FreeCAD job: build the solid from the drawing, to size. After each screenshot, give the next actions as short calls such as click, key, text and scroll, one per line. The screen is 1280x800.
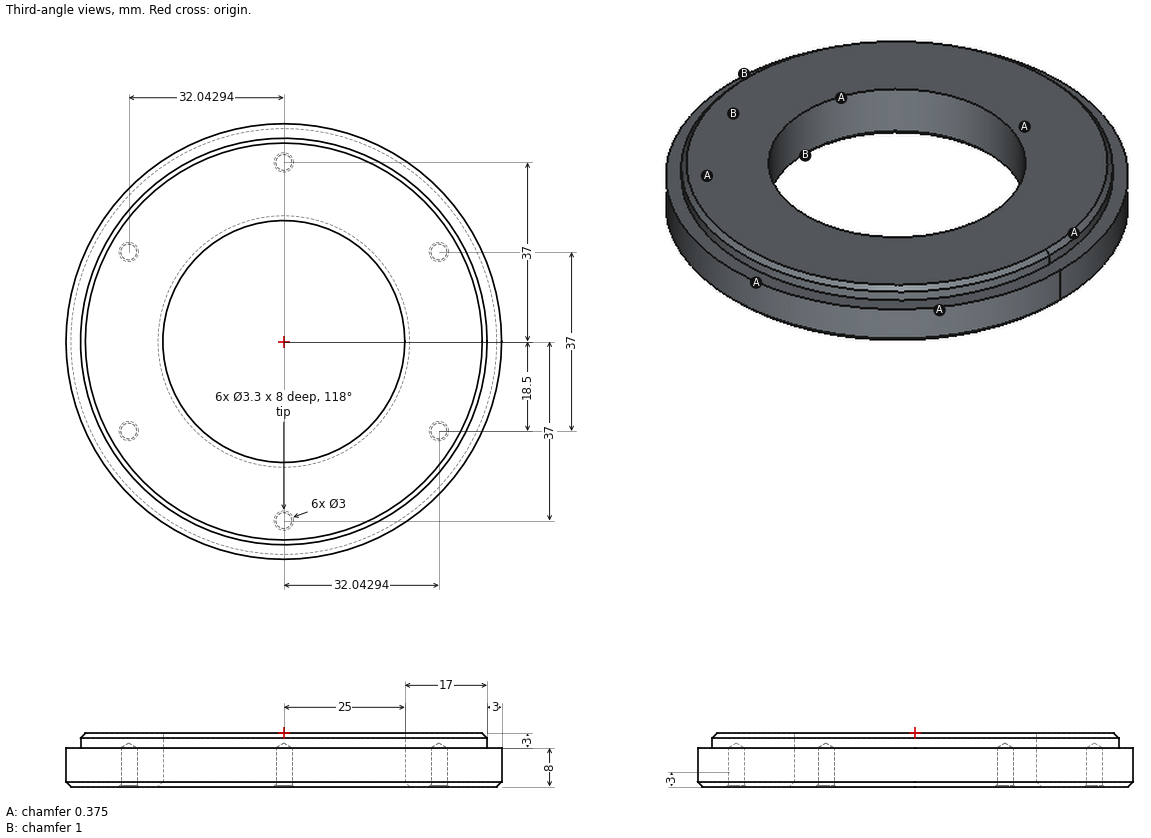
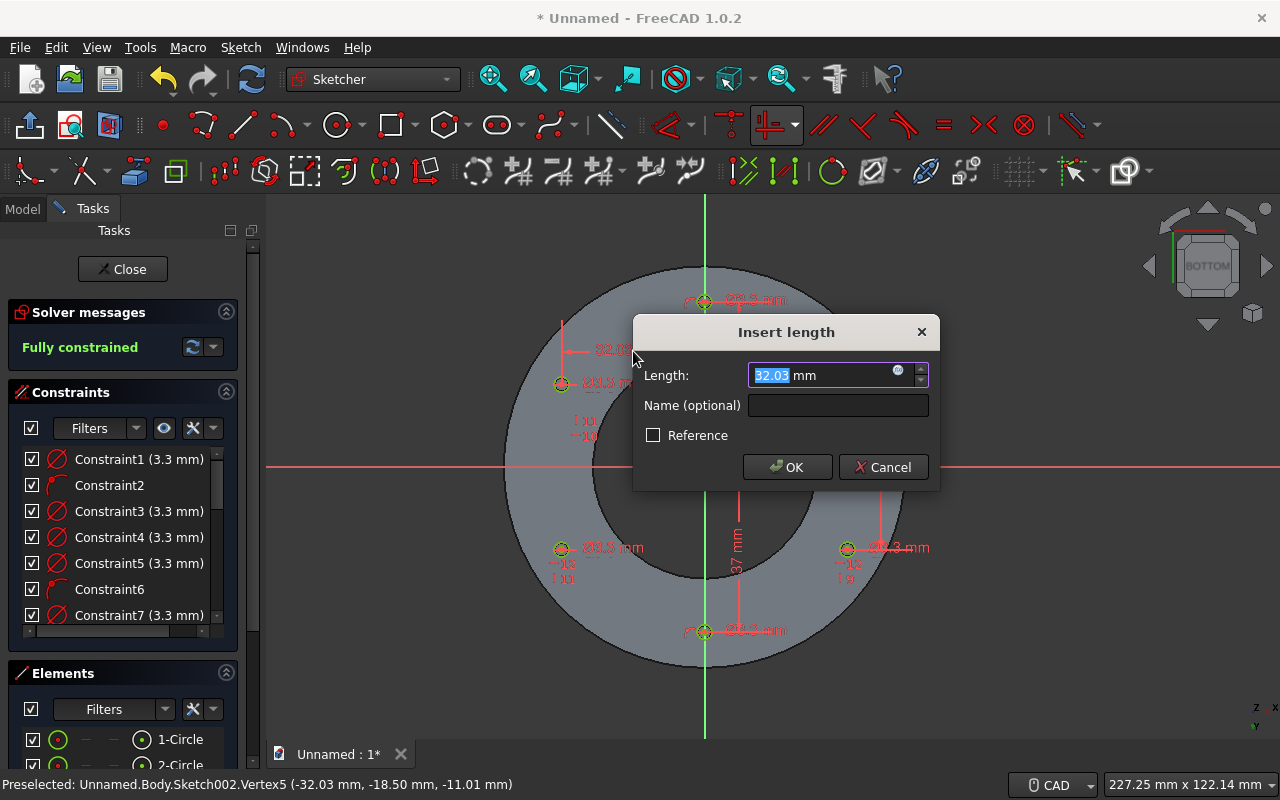
text(32.04294)
key(Return)
key(Escape)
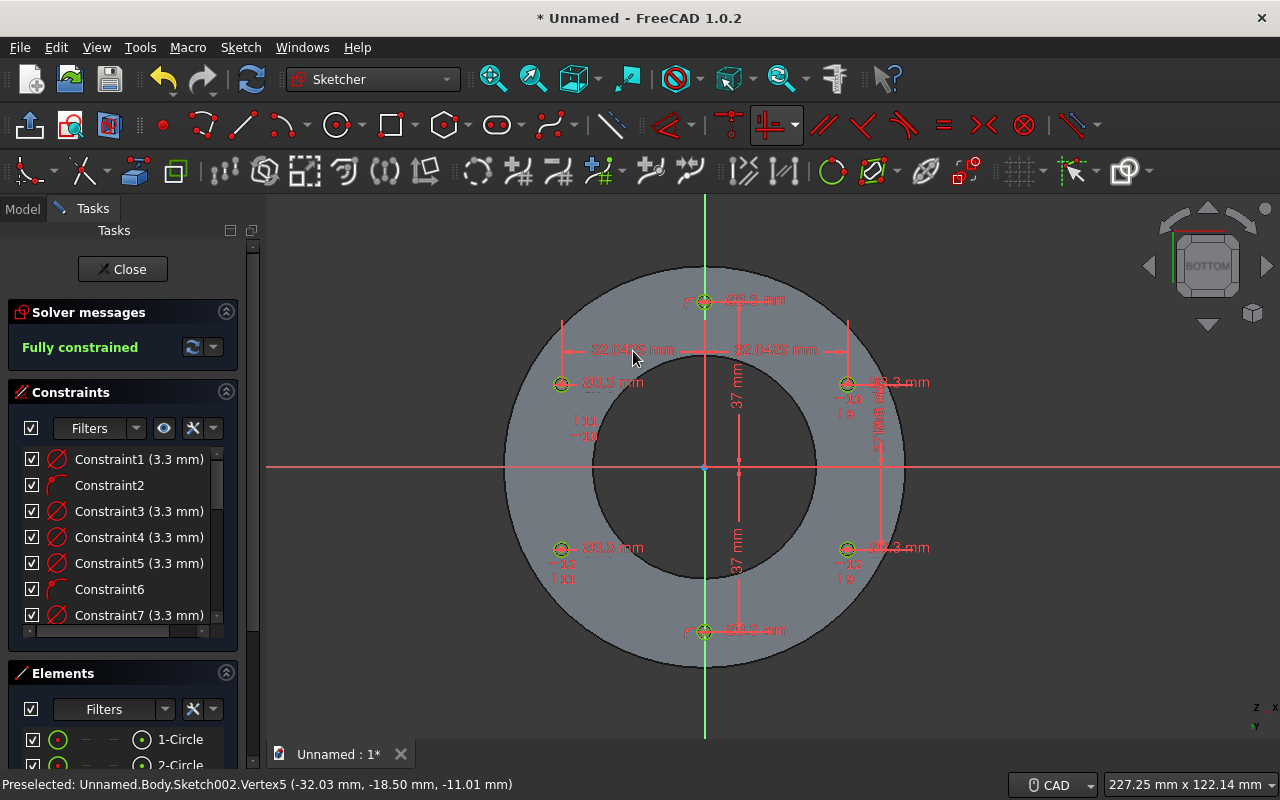
click(123, 269)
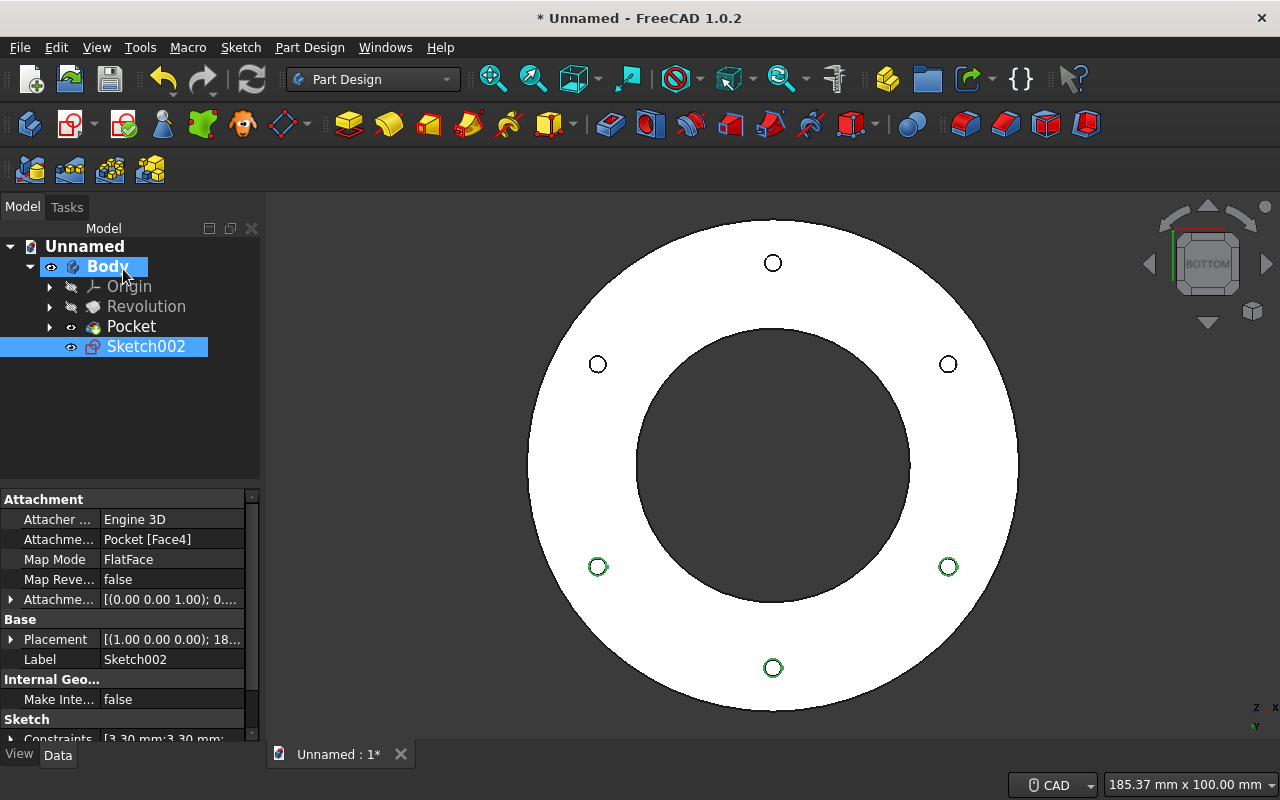
click(652, 124)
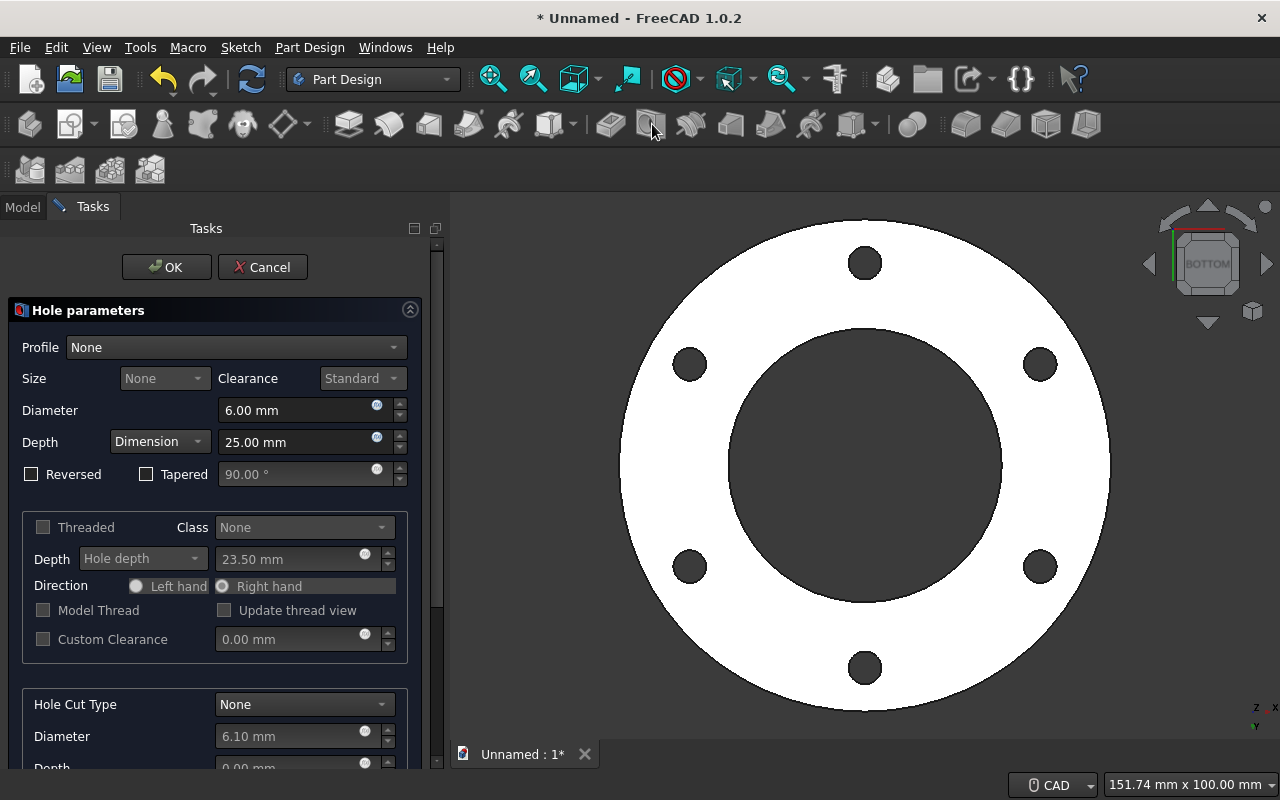
triple_click(305, 410)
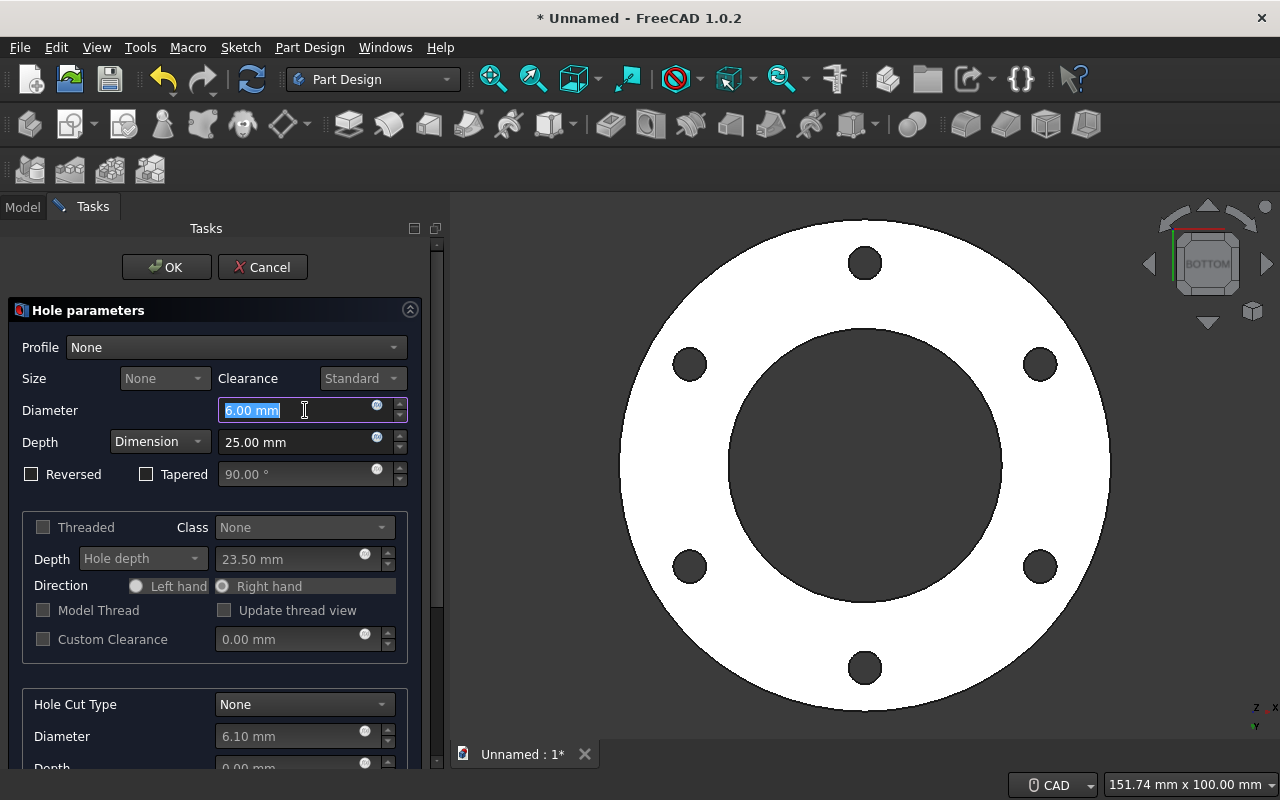
text(3.3)
key(Tab)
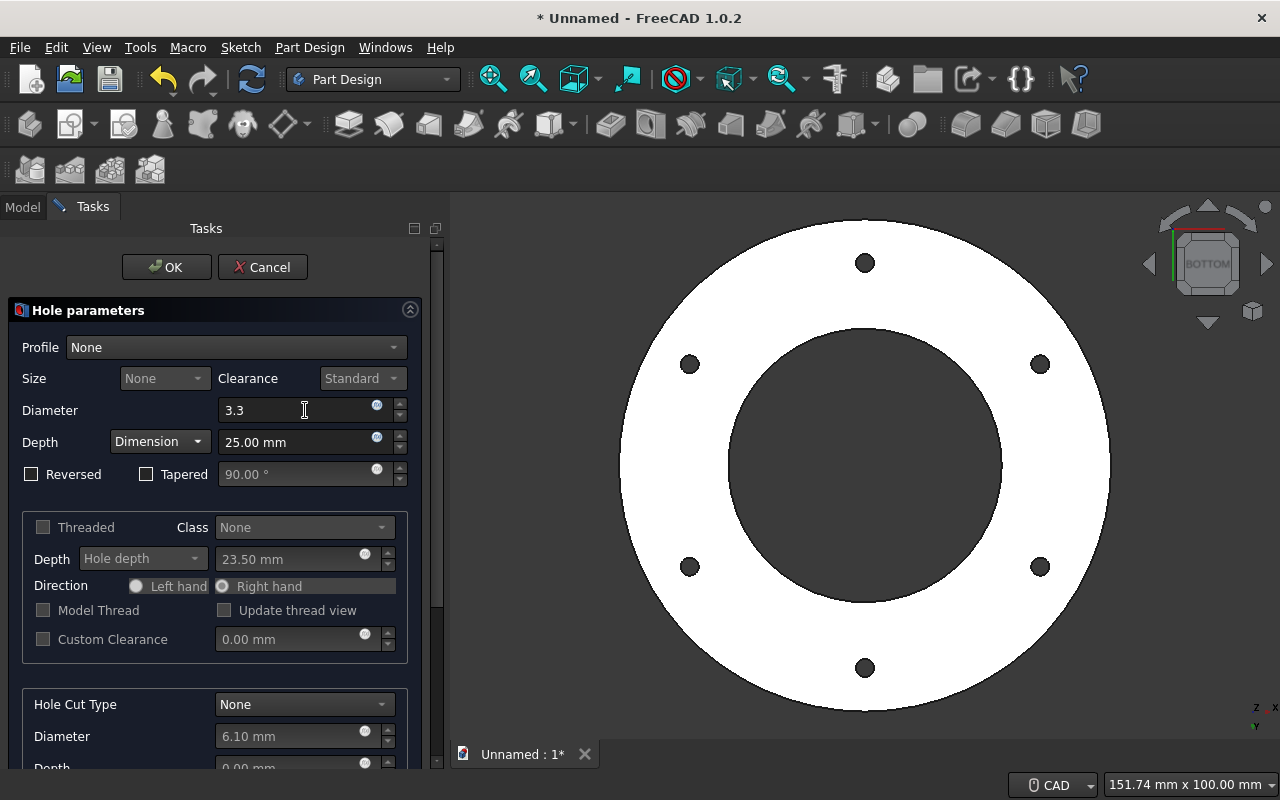
triple_click(305, 442)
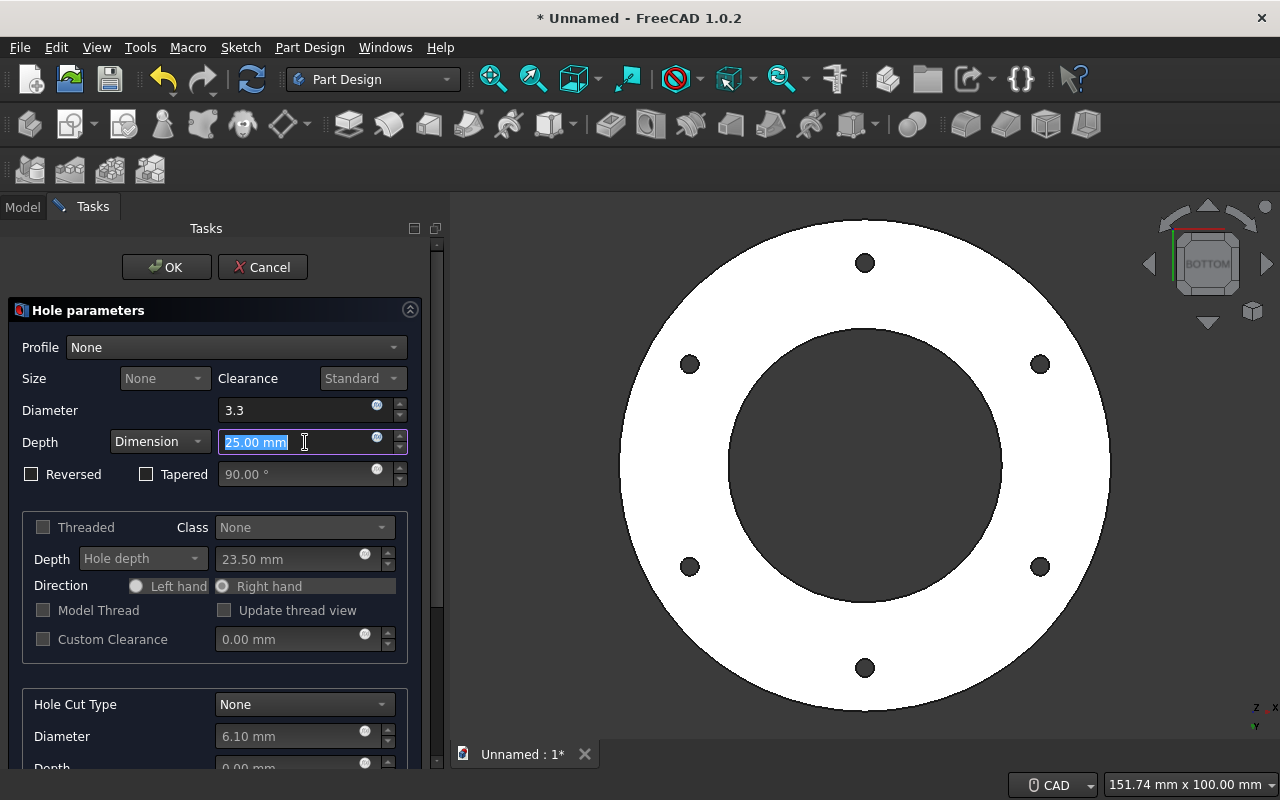
text(8)
key(Tab)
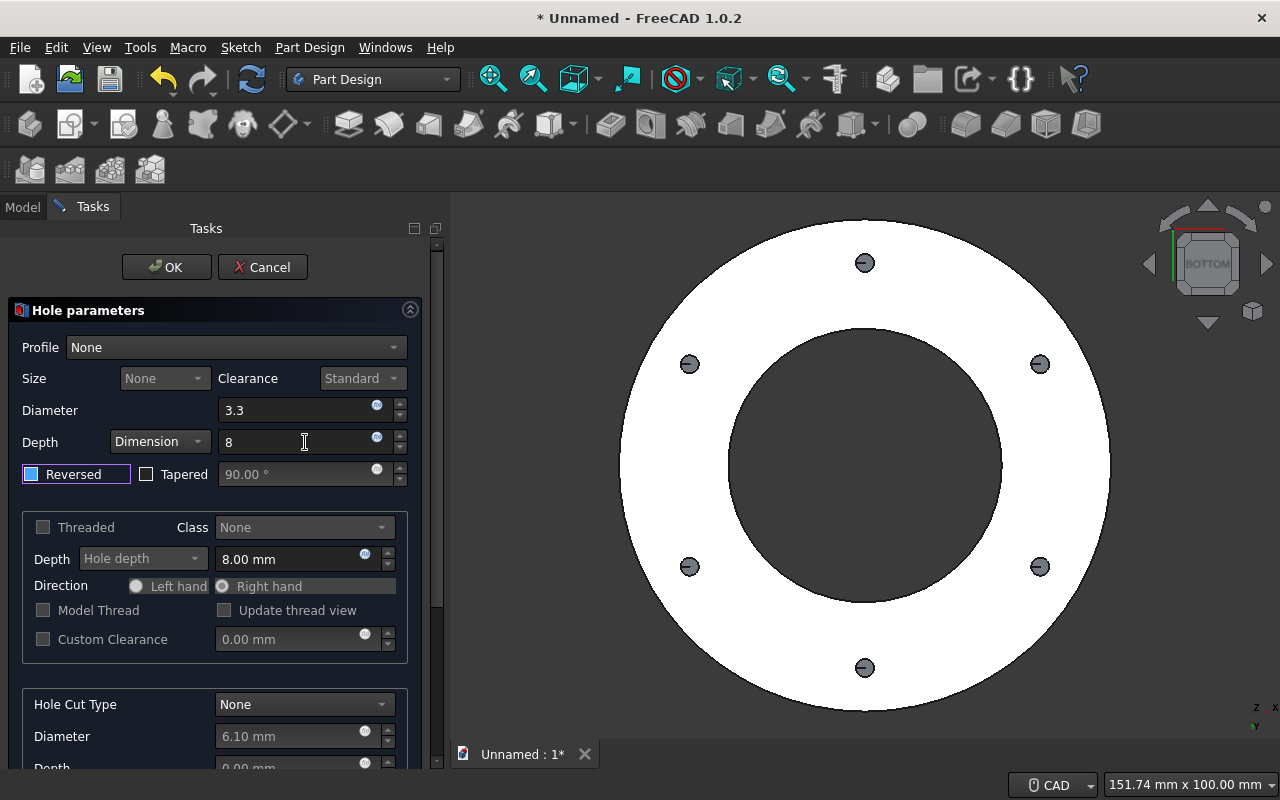
click(167, 267)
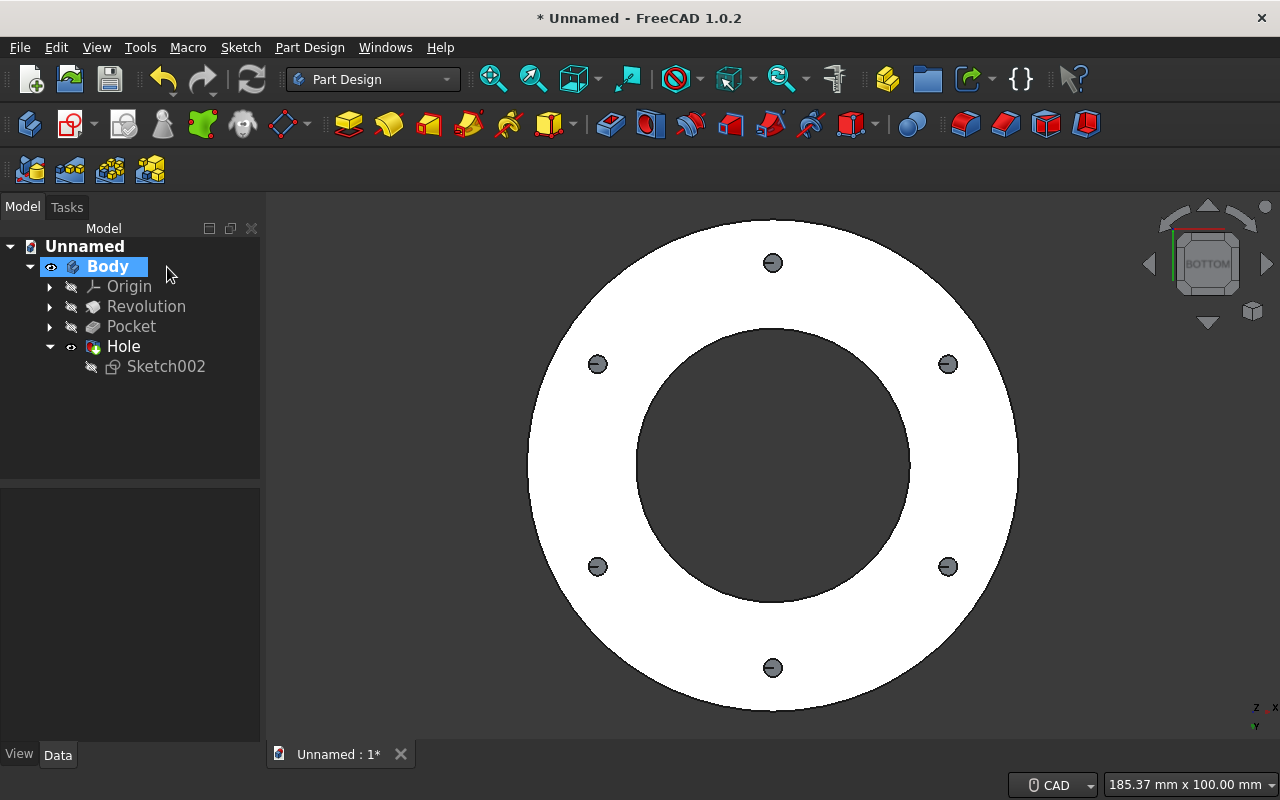
click(607, 566)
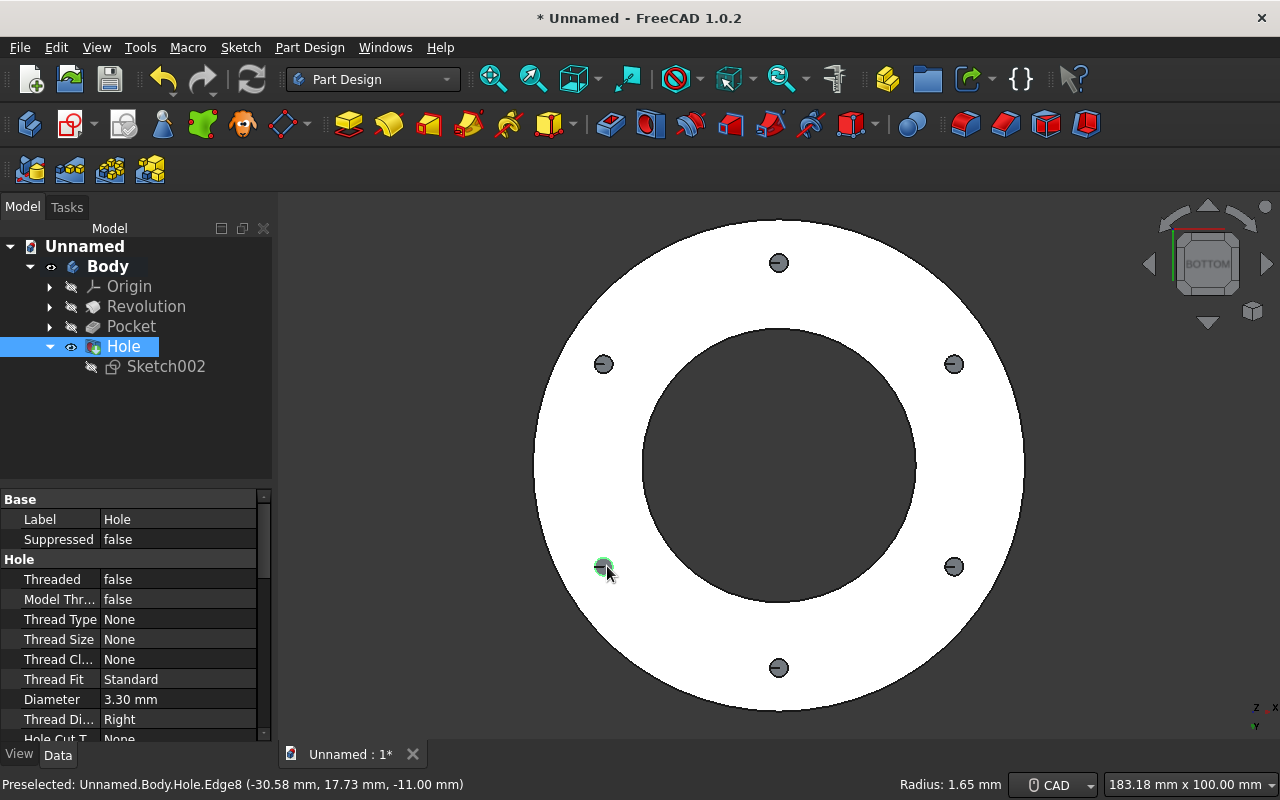
click(613, 363, ctrl)